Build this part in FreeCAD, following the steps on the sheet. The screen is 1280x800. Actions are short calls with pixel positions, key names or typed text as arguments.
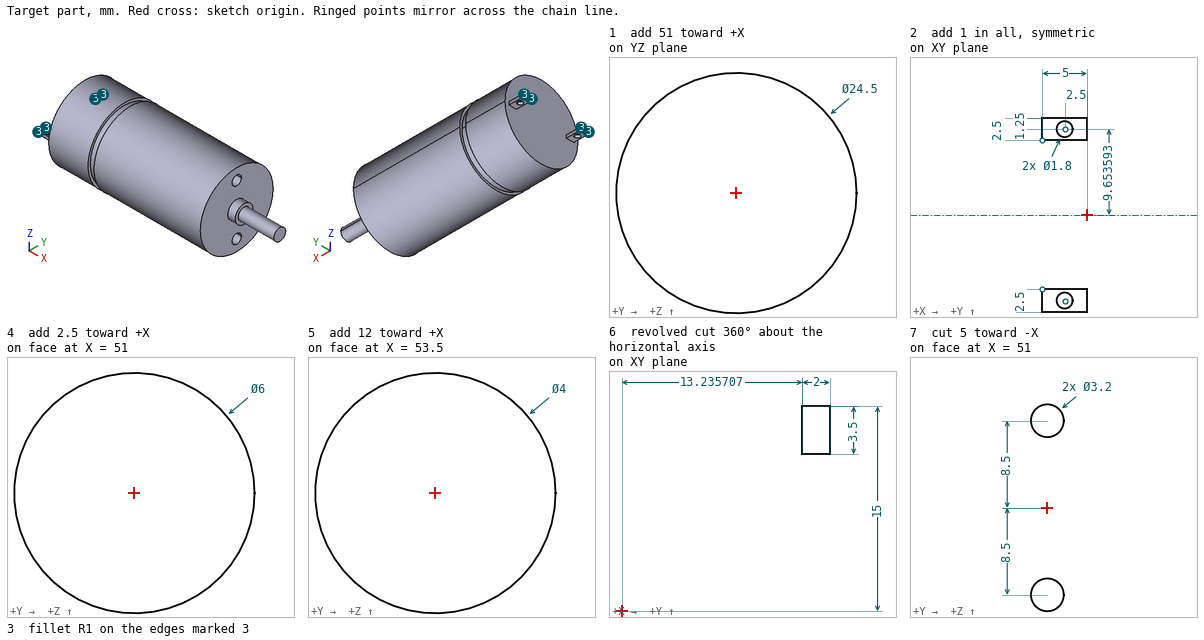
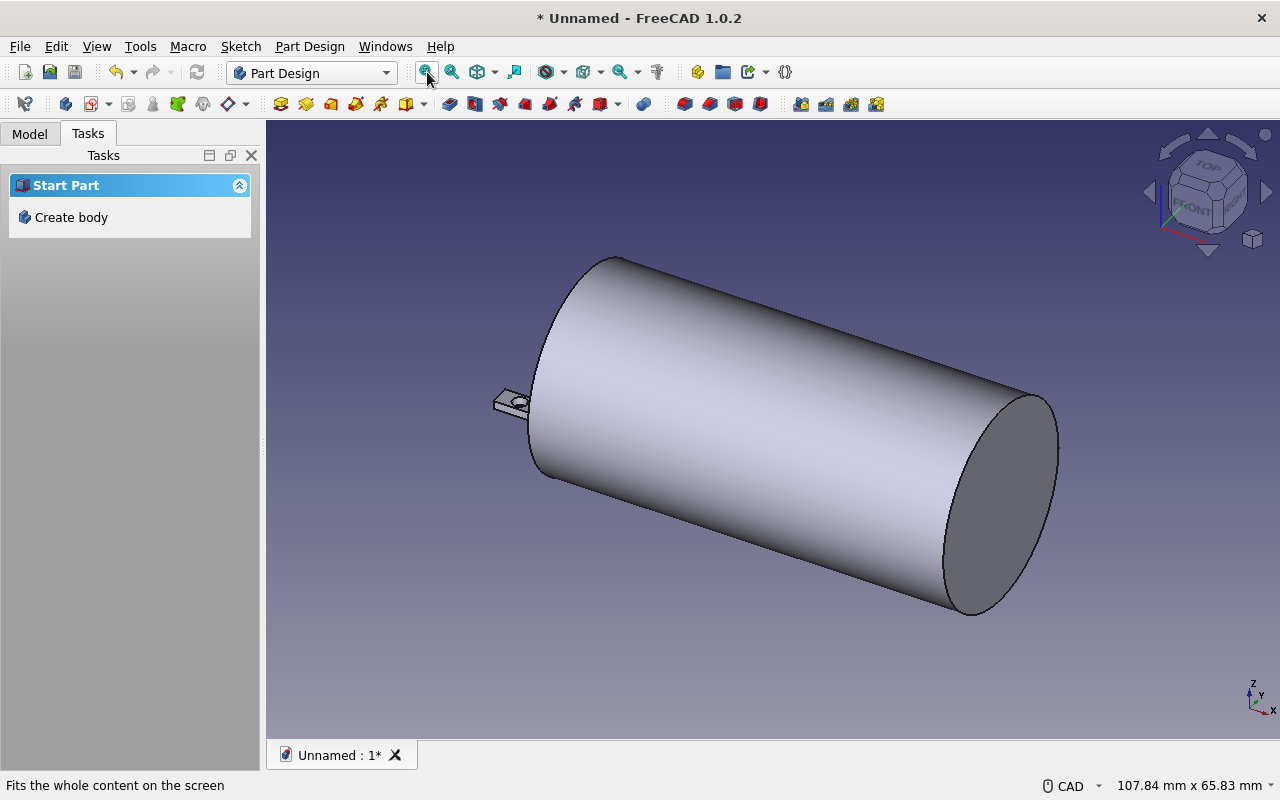
key(0)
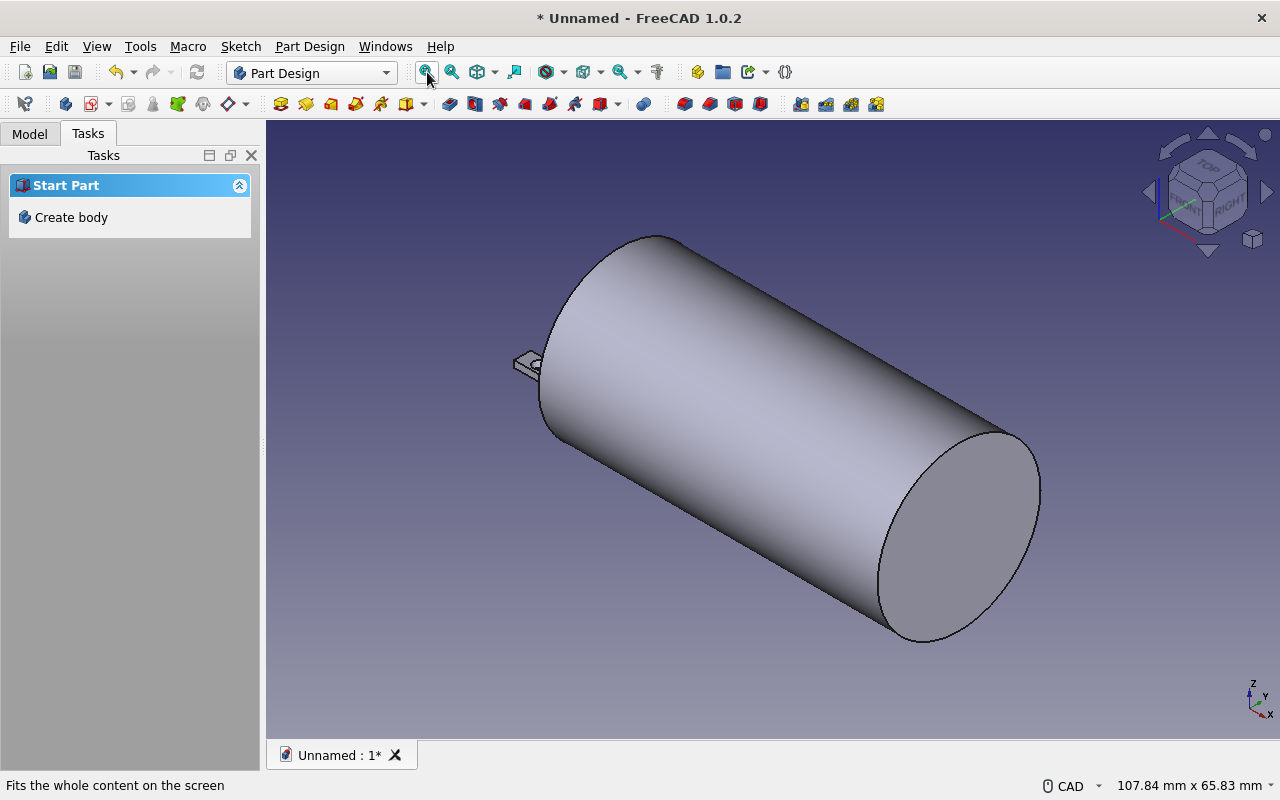
scroll(643, 289, up, 8)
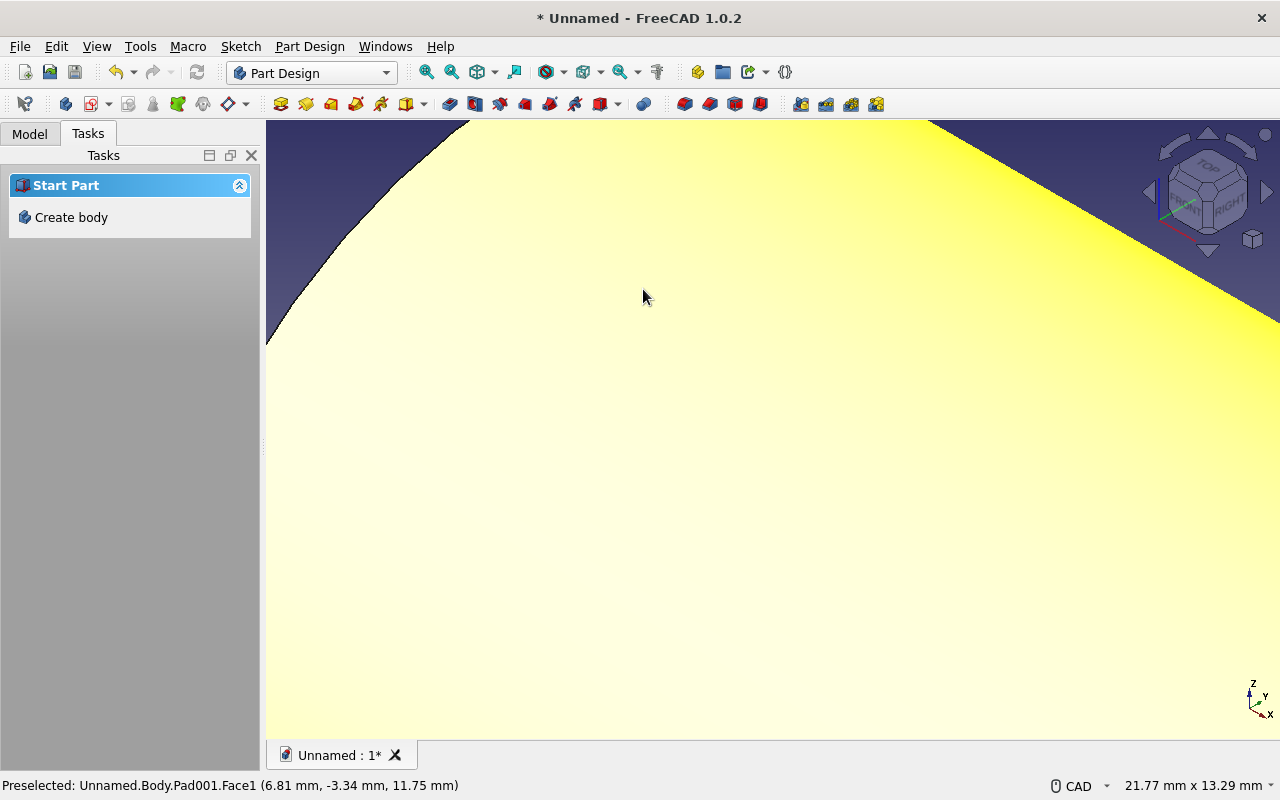
click(427, 72)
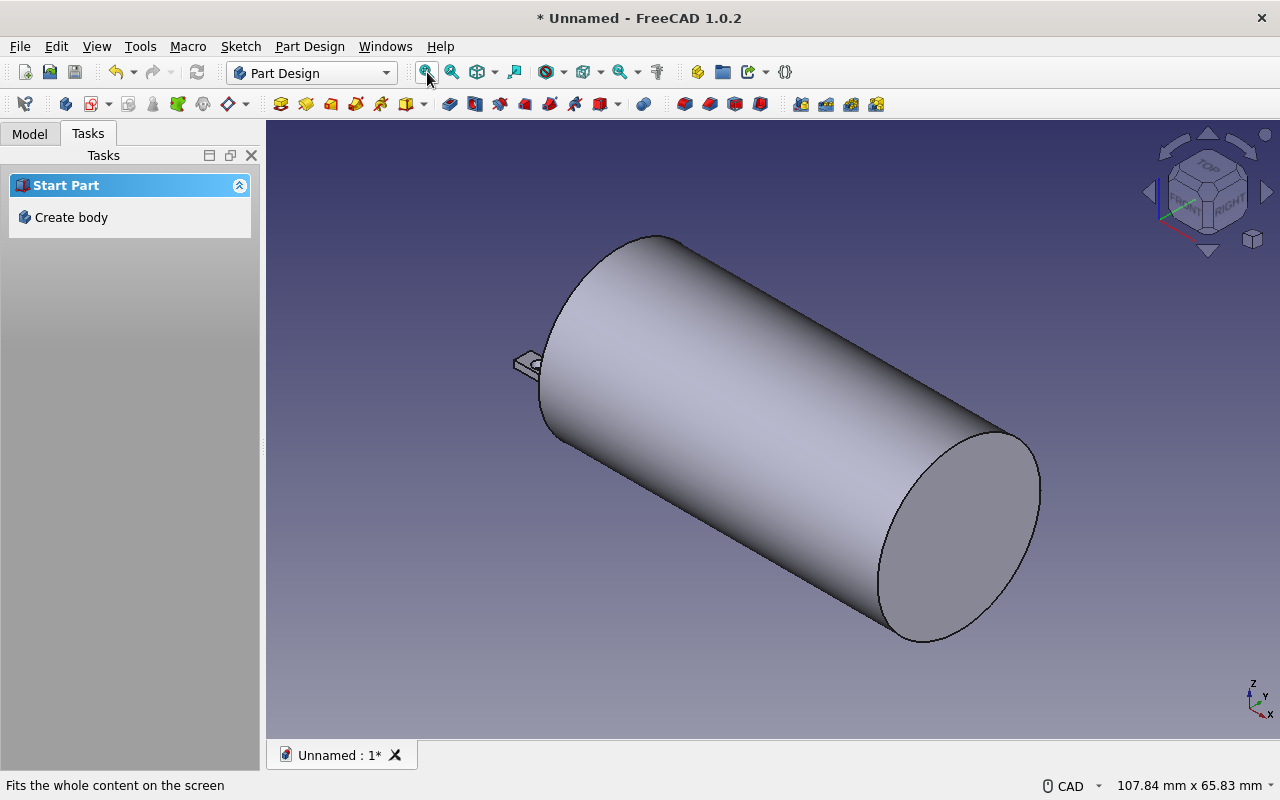
key(2)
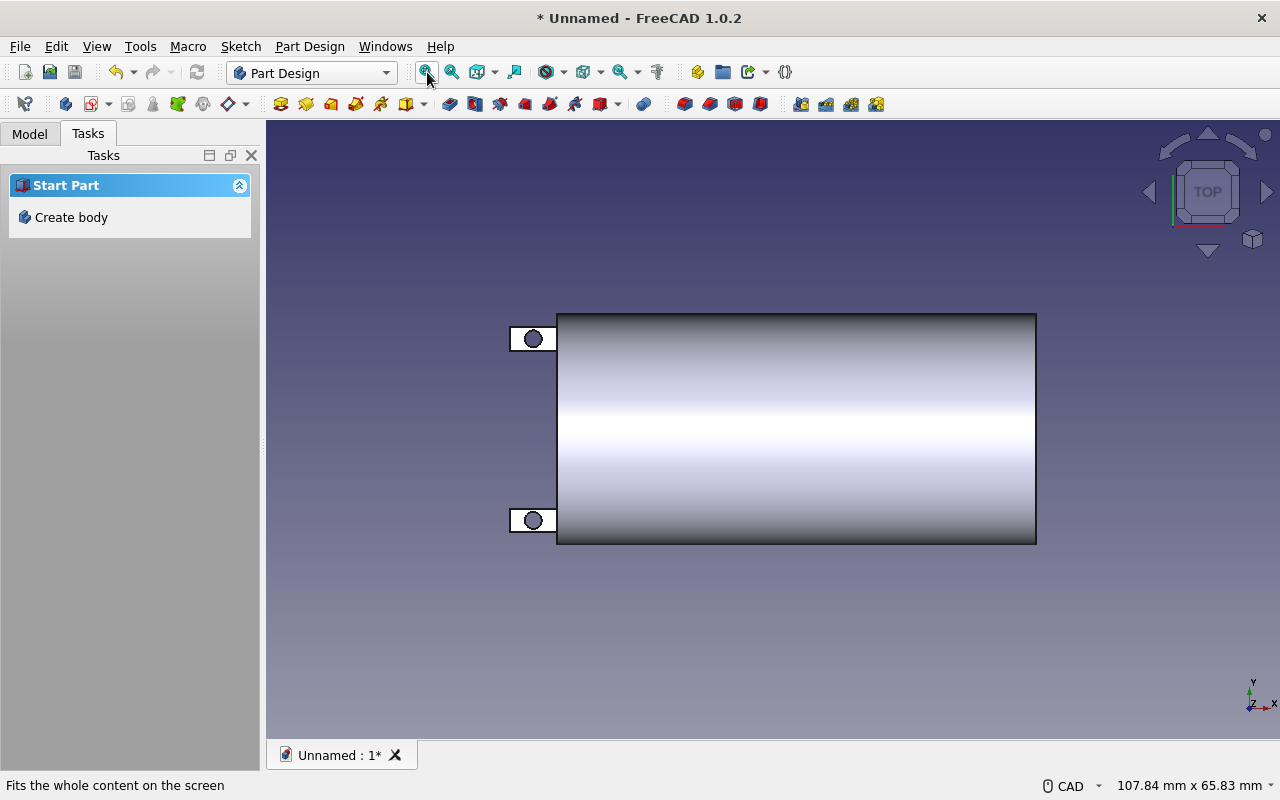
scroll(510, 350, up, 8)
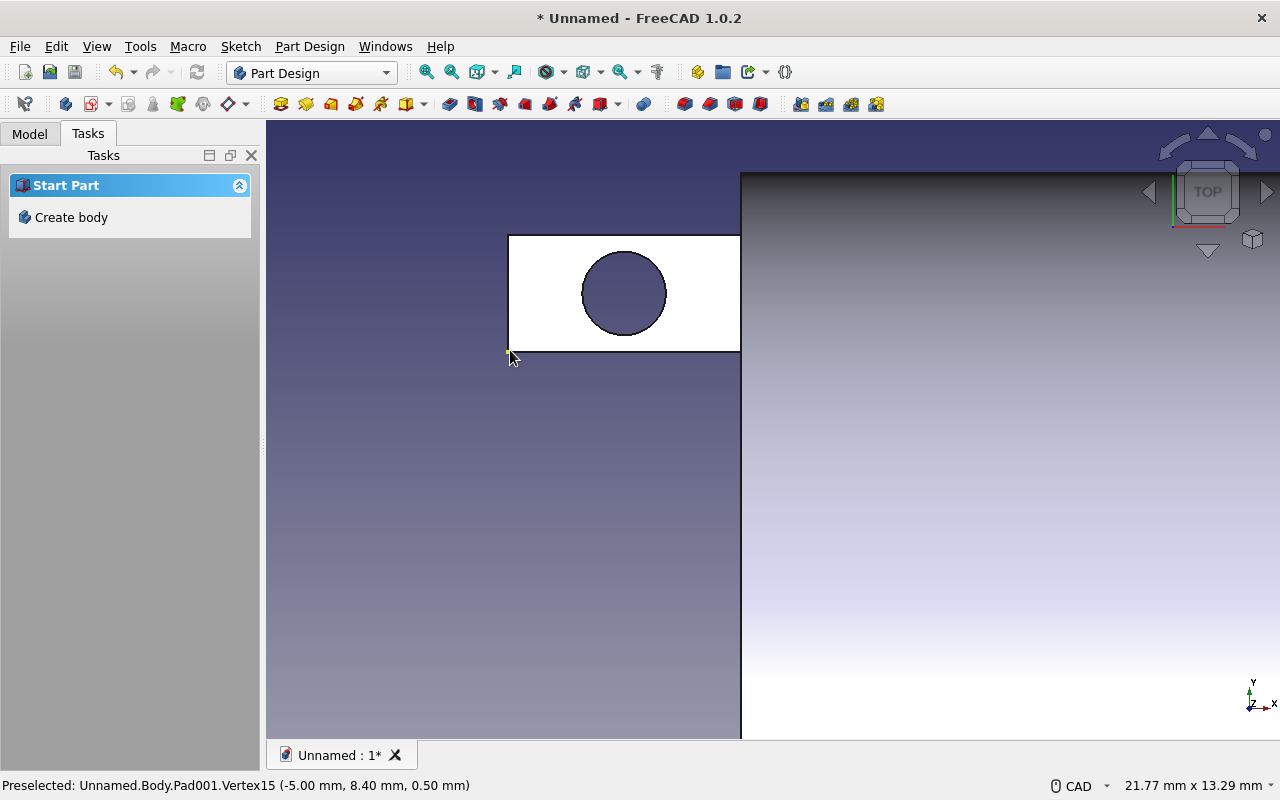
click(427, 72)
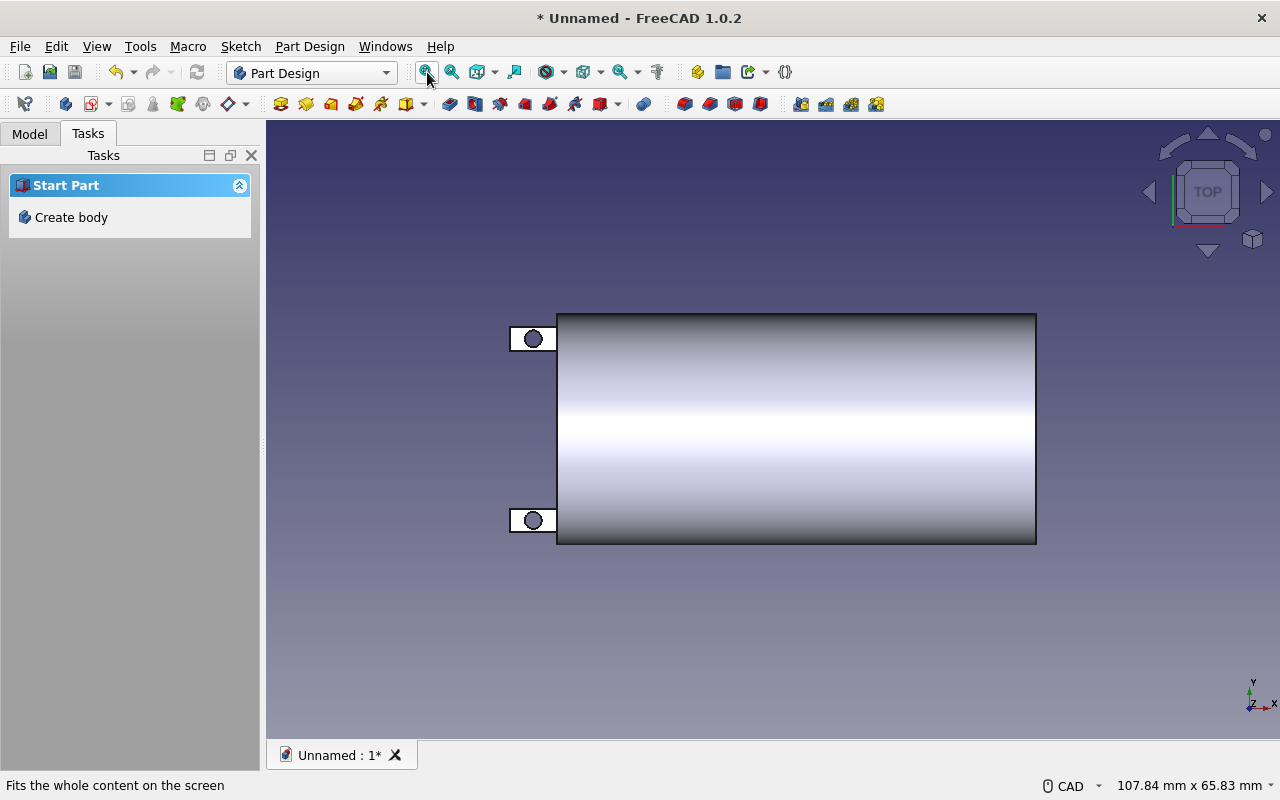
key(1)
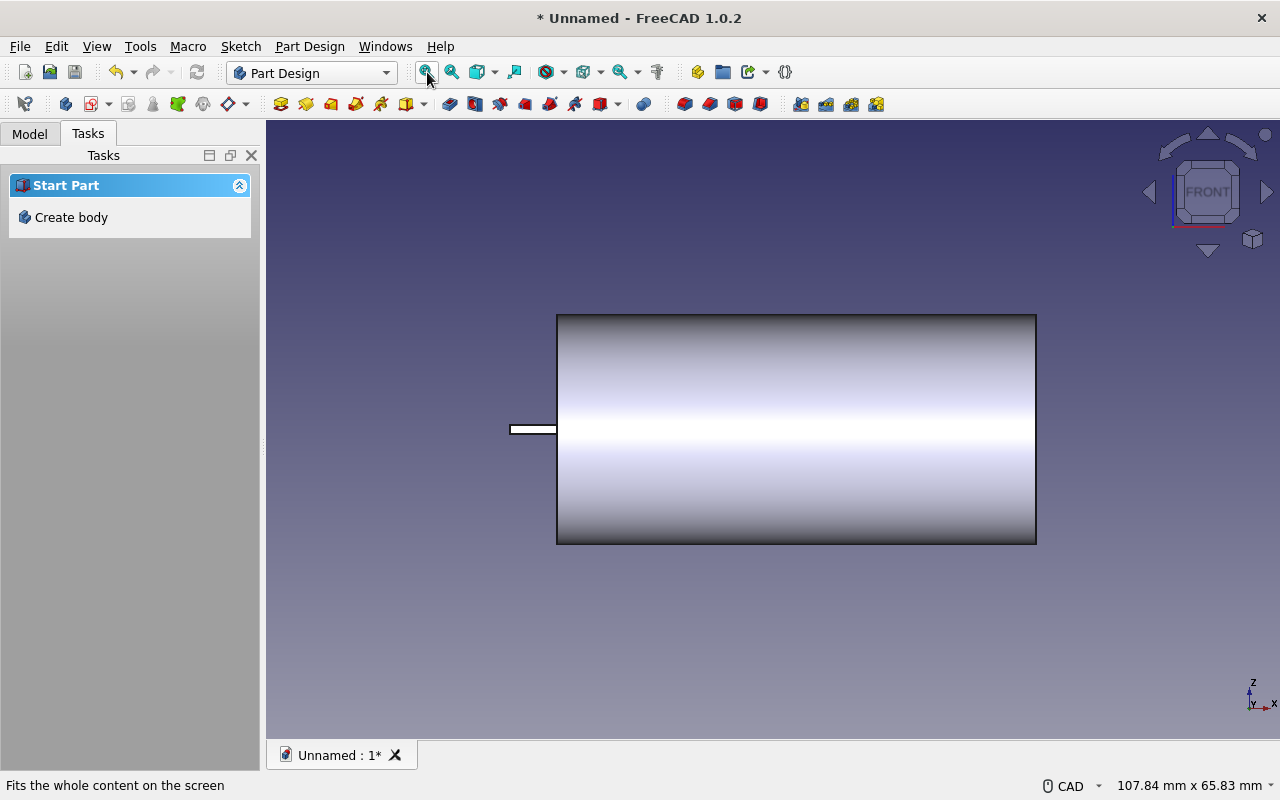
scroll(510, 428, up, 8)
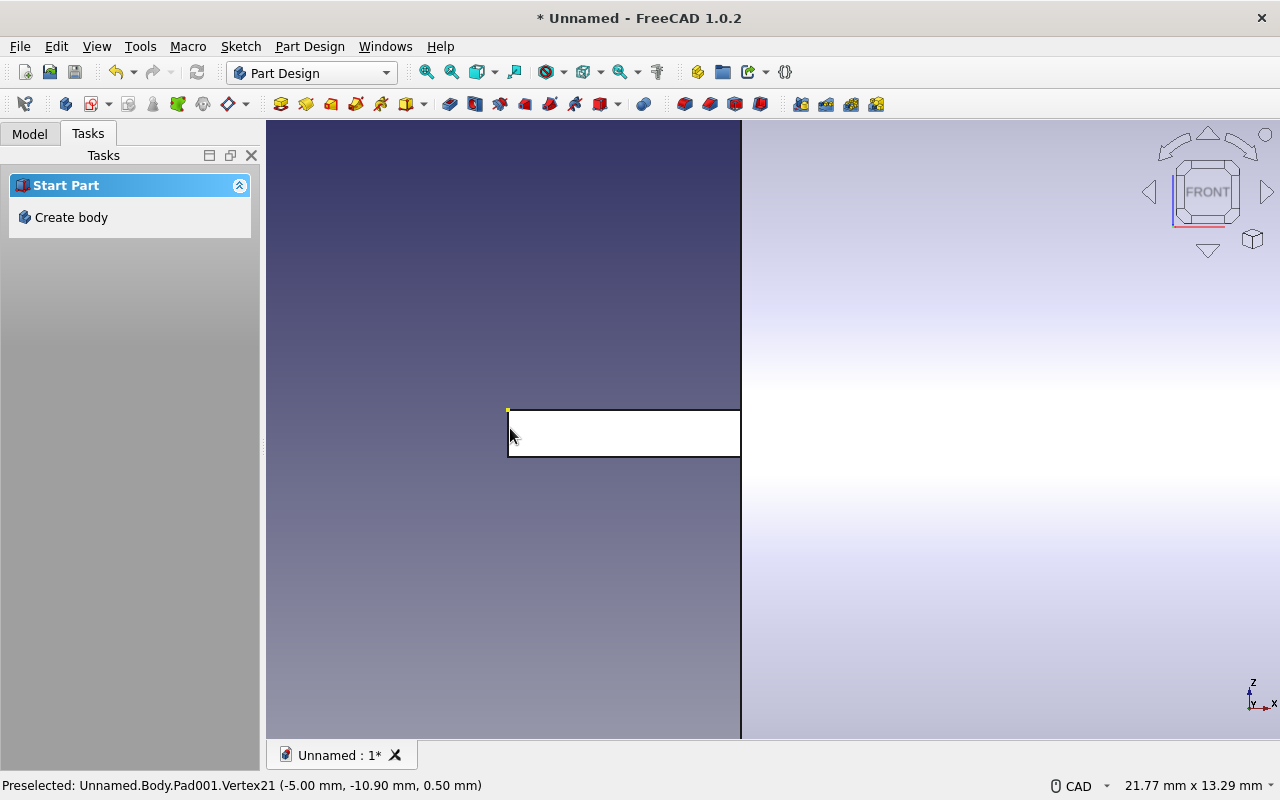
click(508, 432)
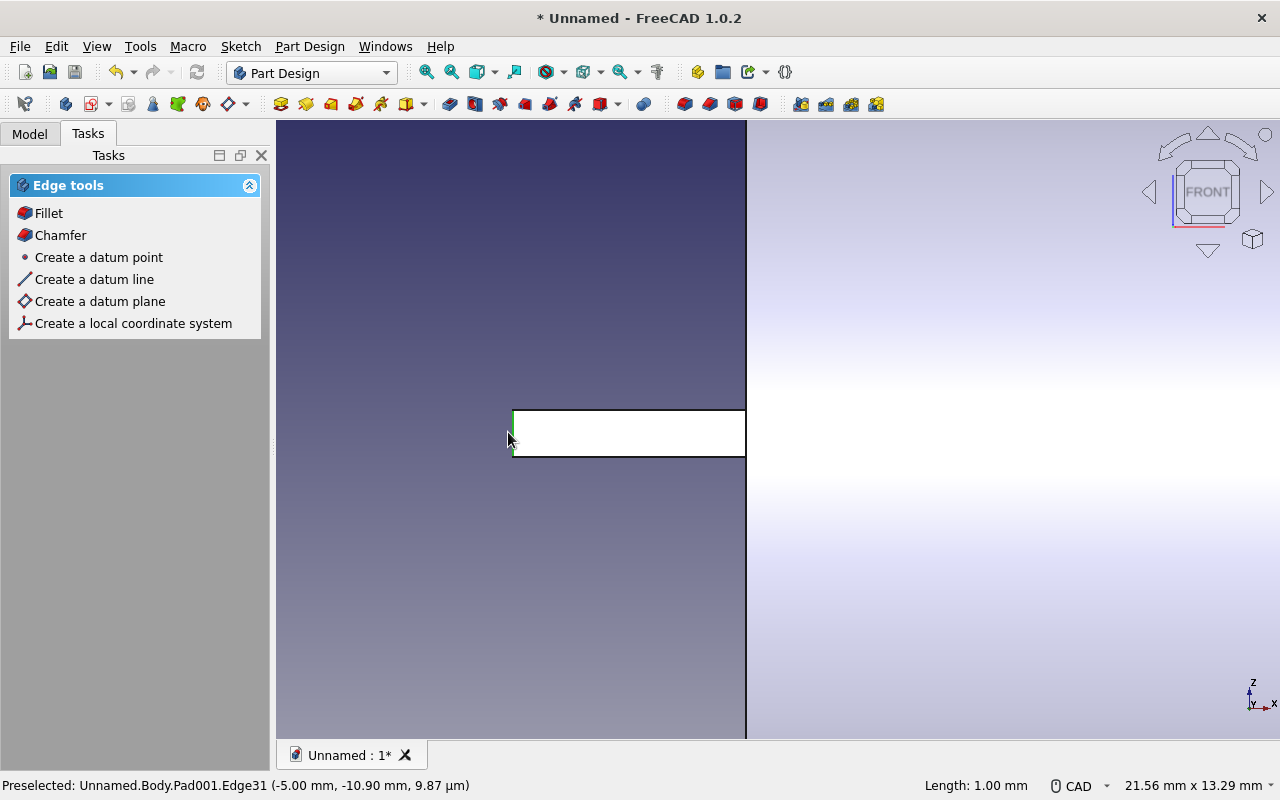
click(427, 72)